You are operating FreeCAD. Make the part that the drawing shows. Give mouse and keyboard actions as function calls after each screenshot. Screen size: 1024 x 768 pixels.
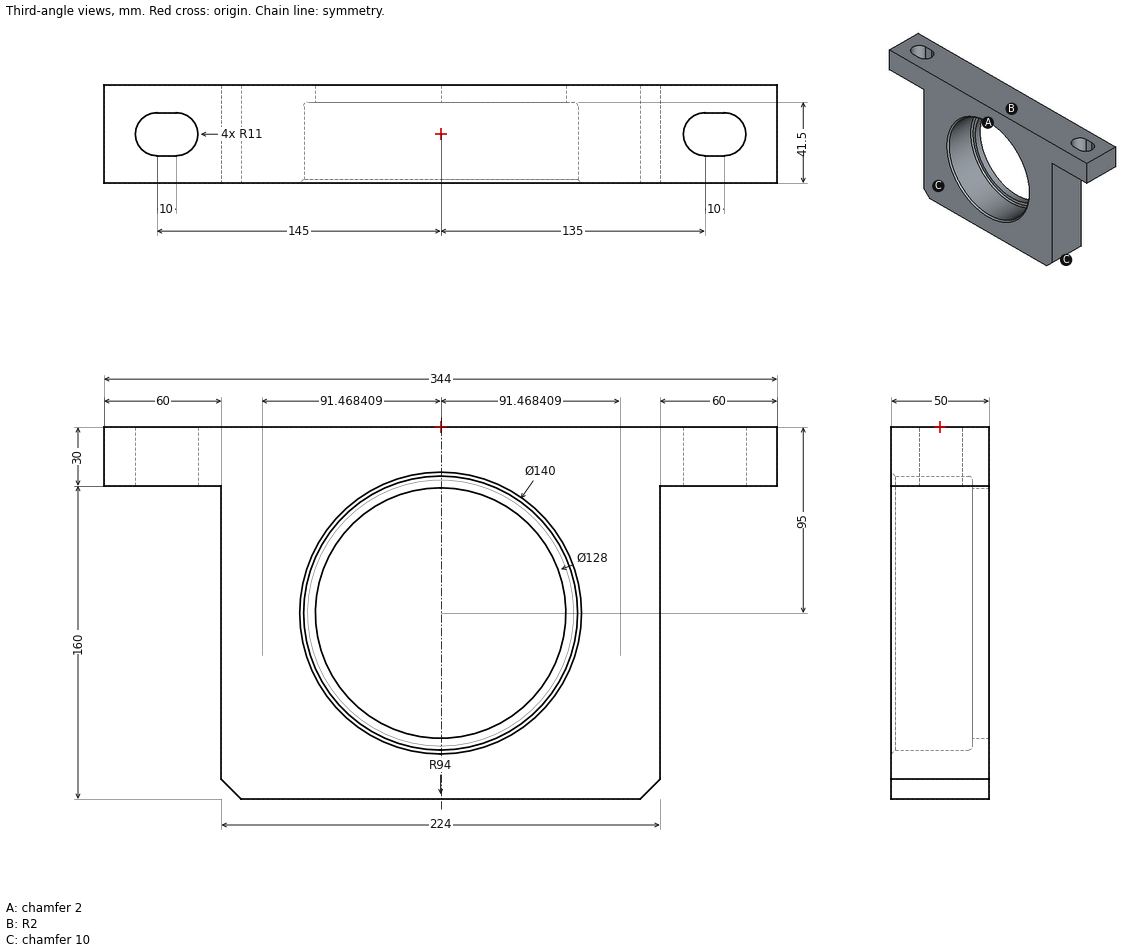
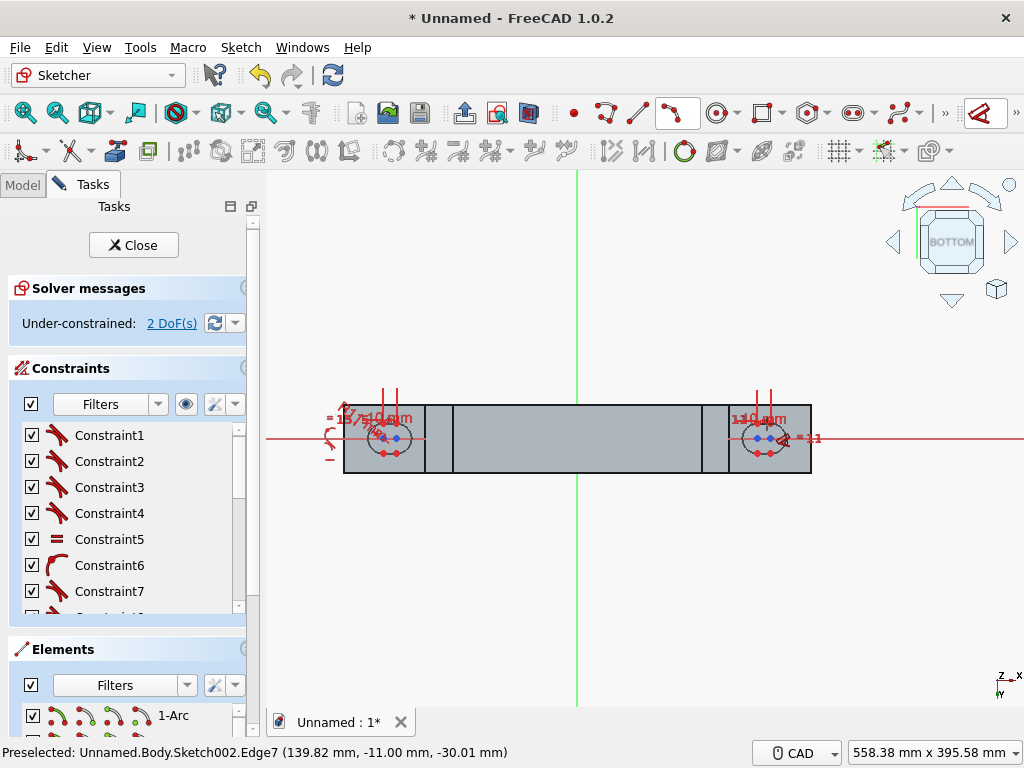
click(383, 424)
click(480, 390)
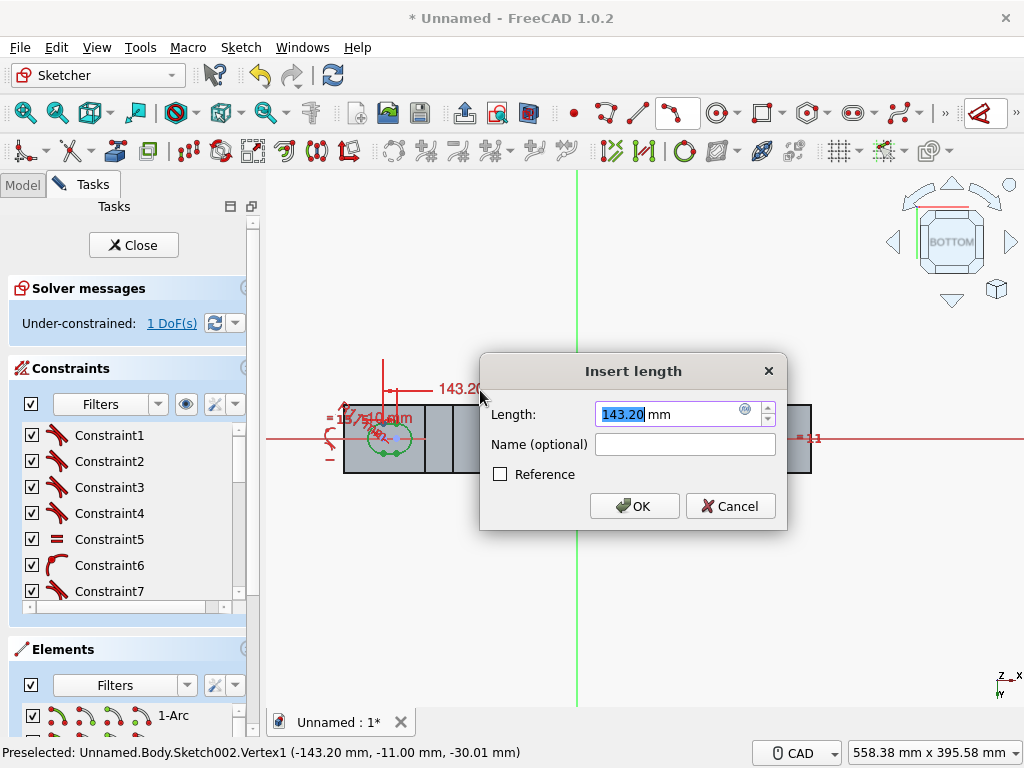
text(145)
key(Return)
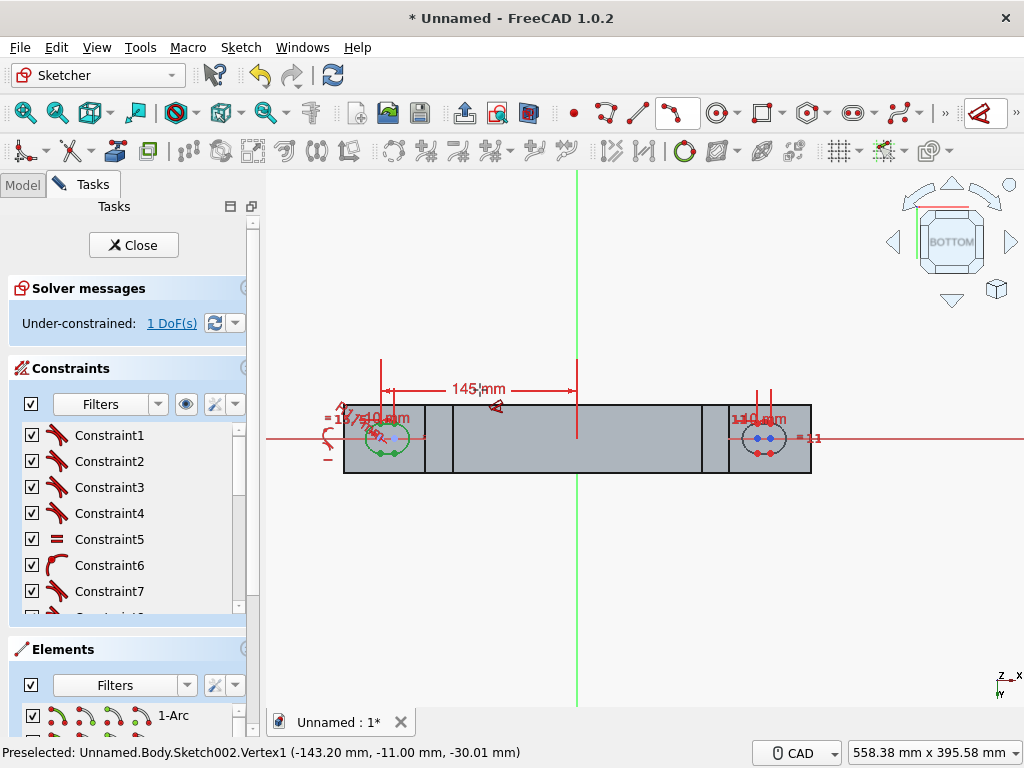
click(757, 424)
click(667, 390)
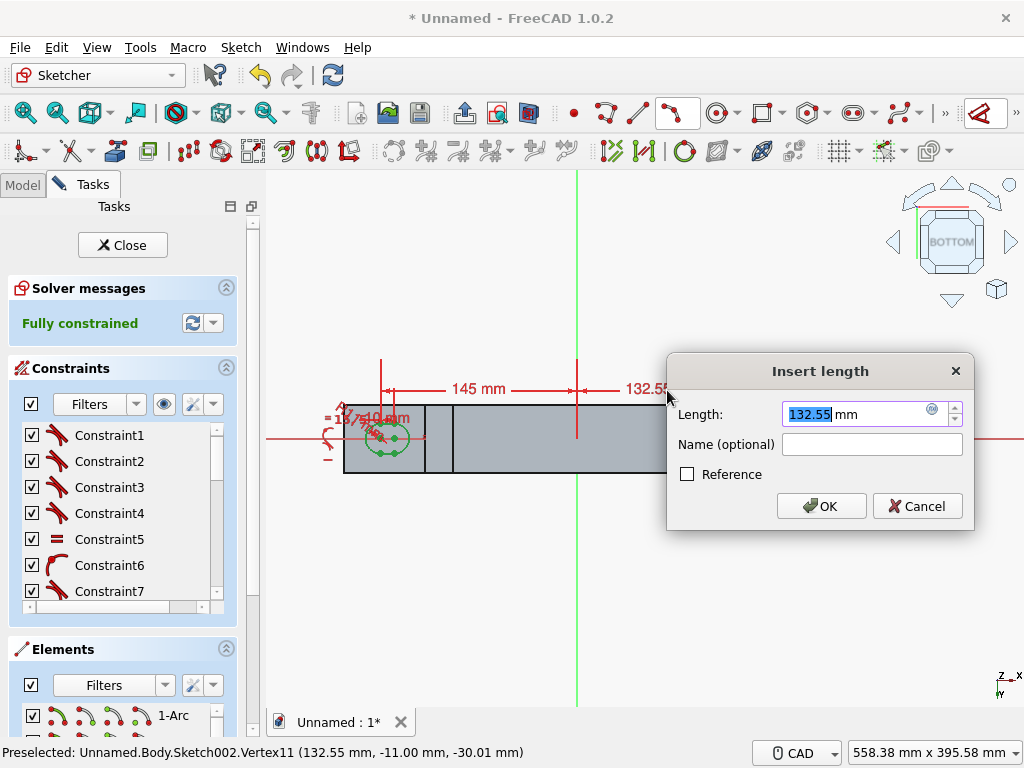
text(135)
key(Return)
key(Escape)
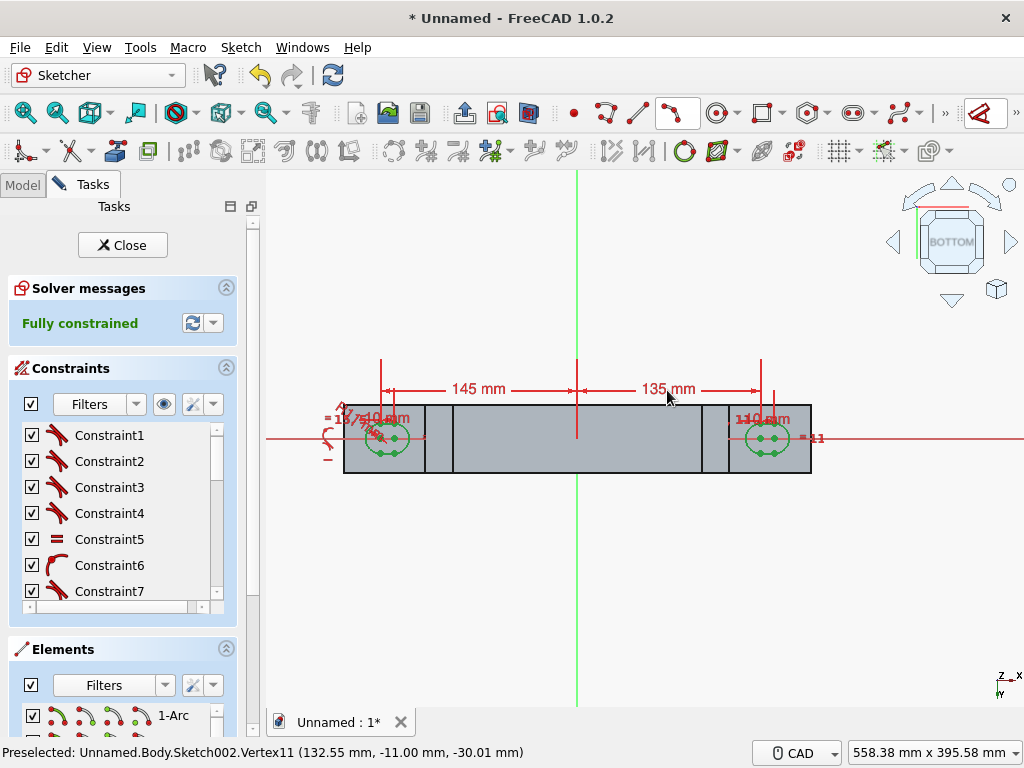
click(123, 245)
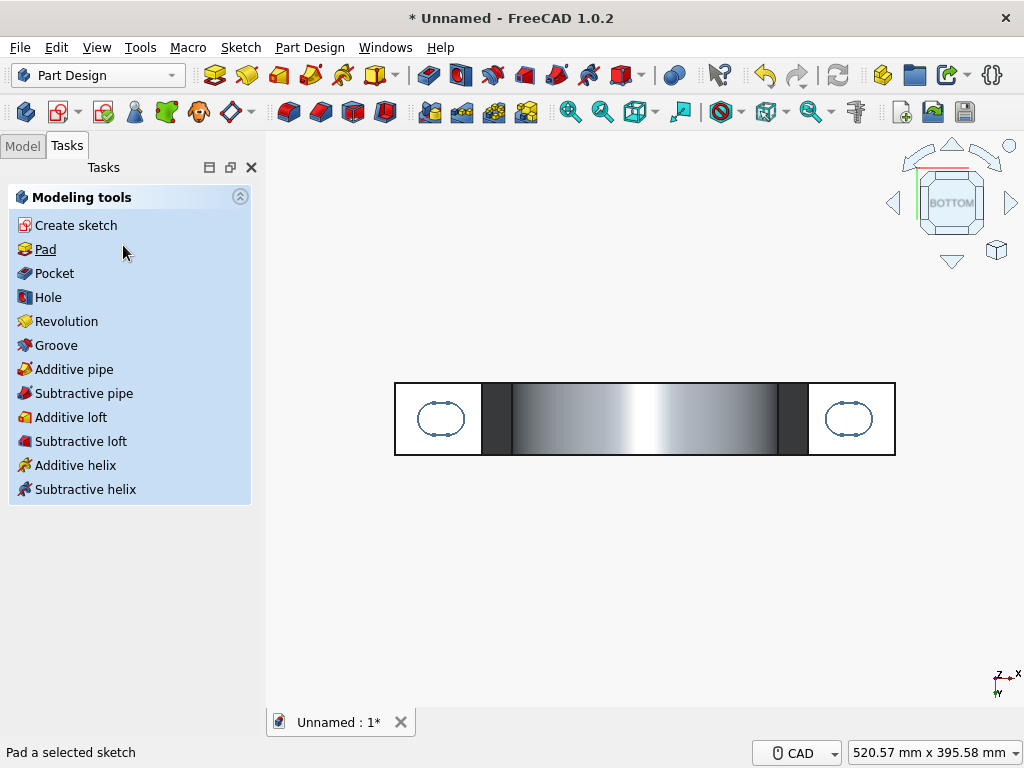
click(430, 76)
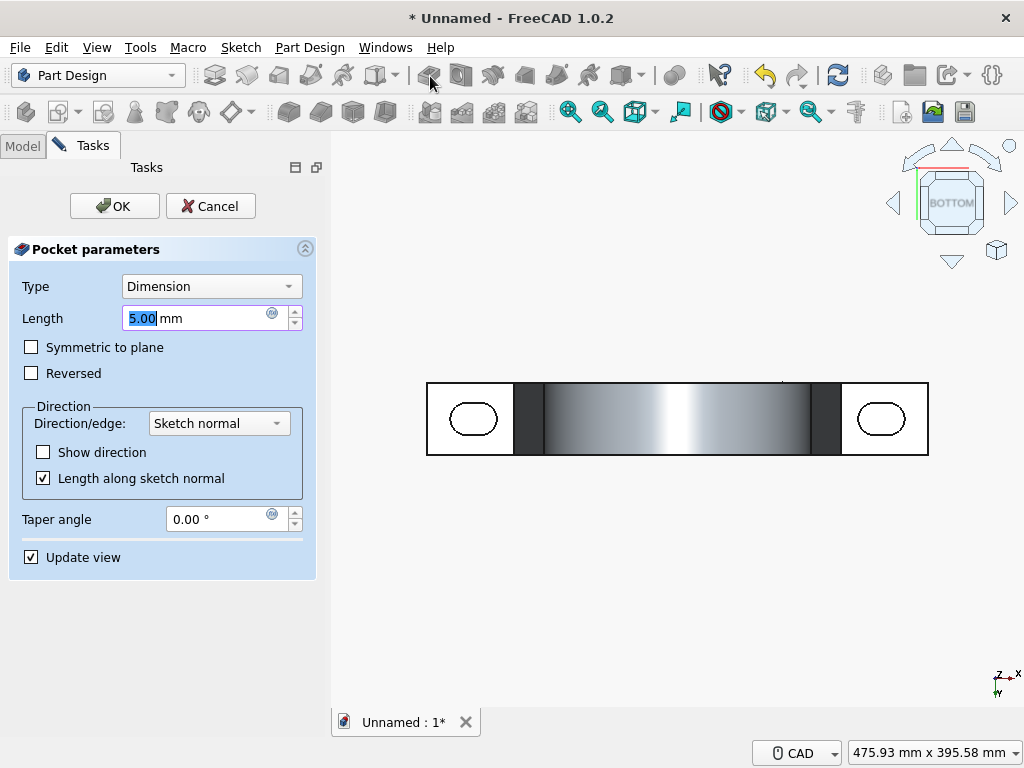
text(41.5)
key(Tab)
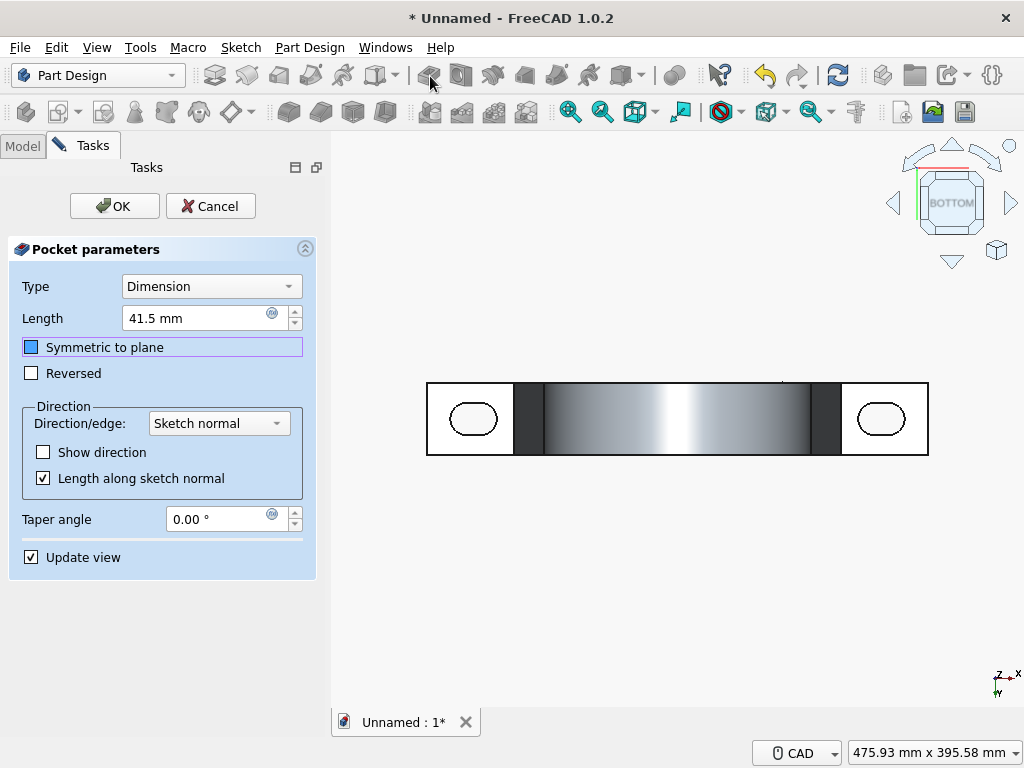
click(115, 206)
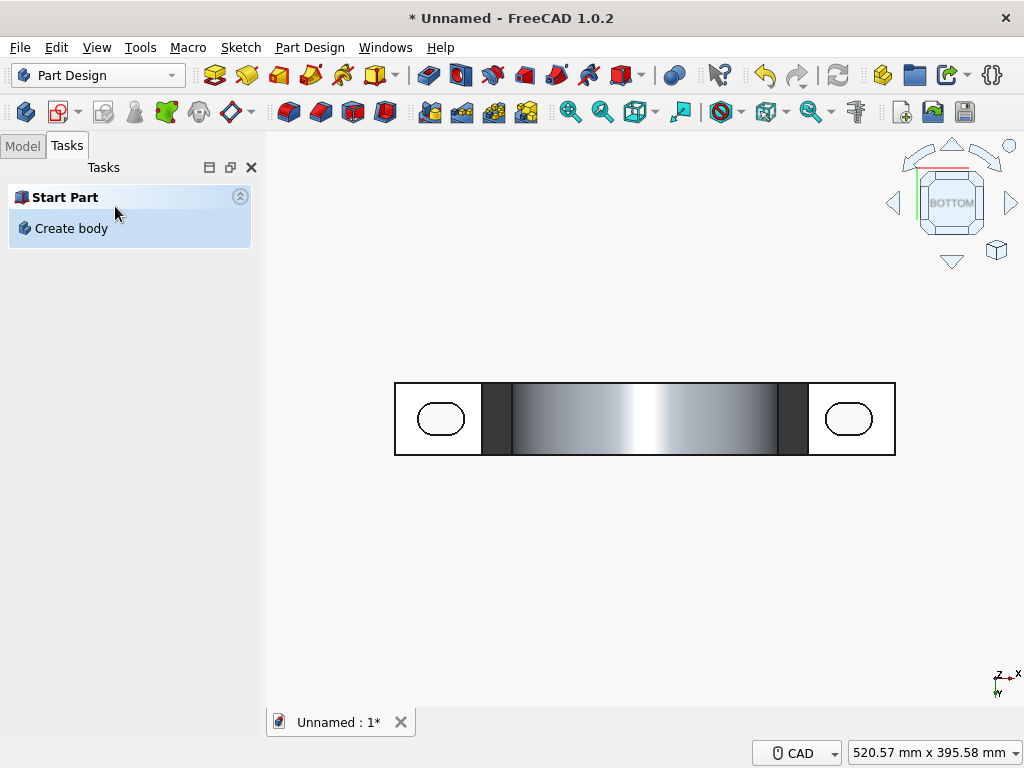
key(4)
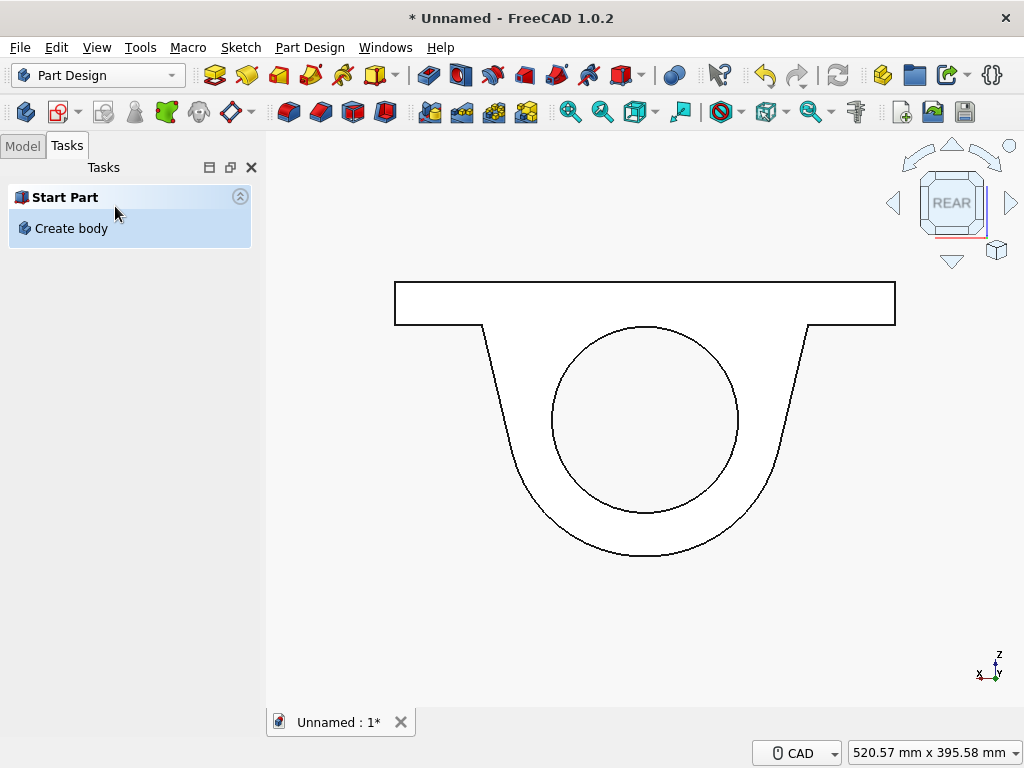
click(430, 300)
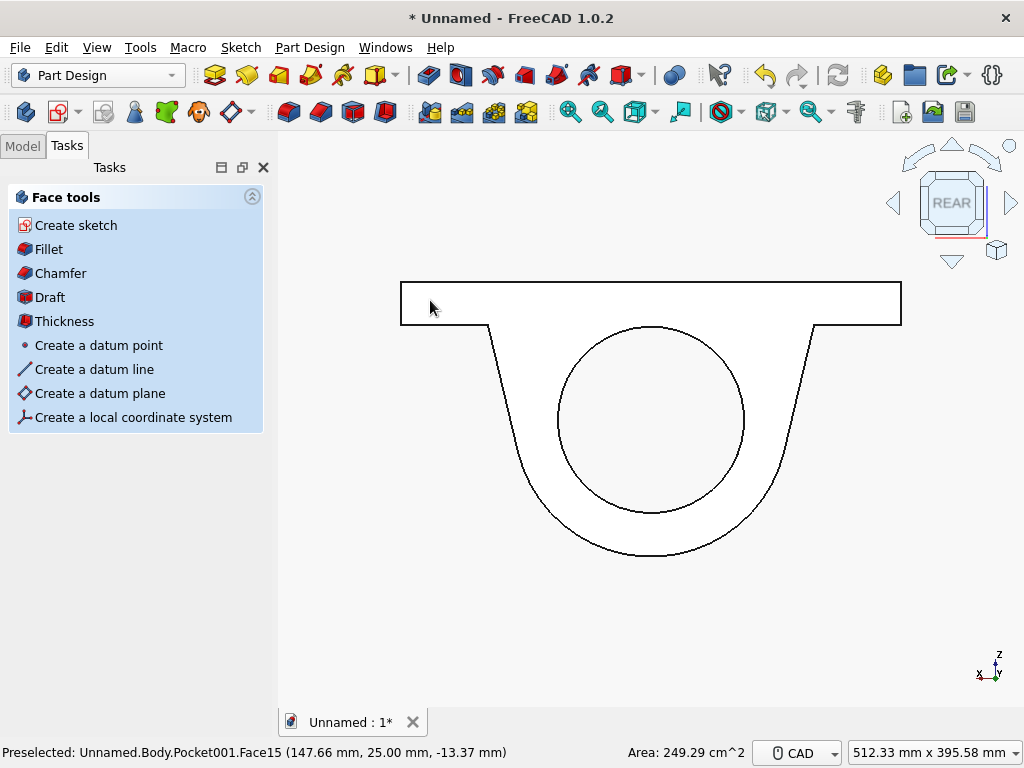
click(58, 112)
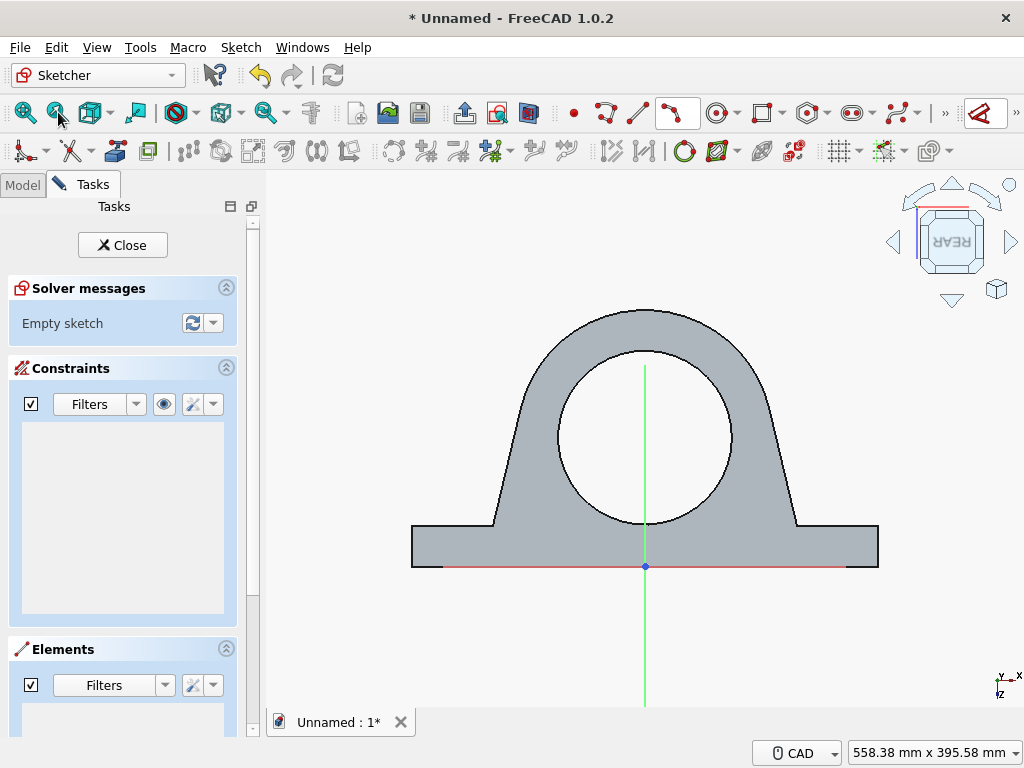
key(g)
key(m)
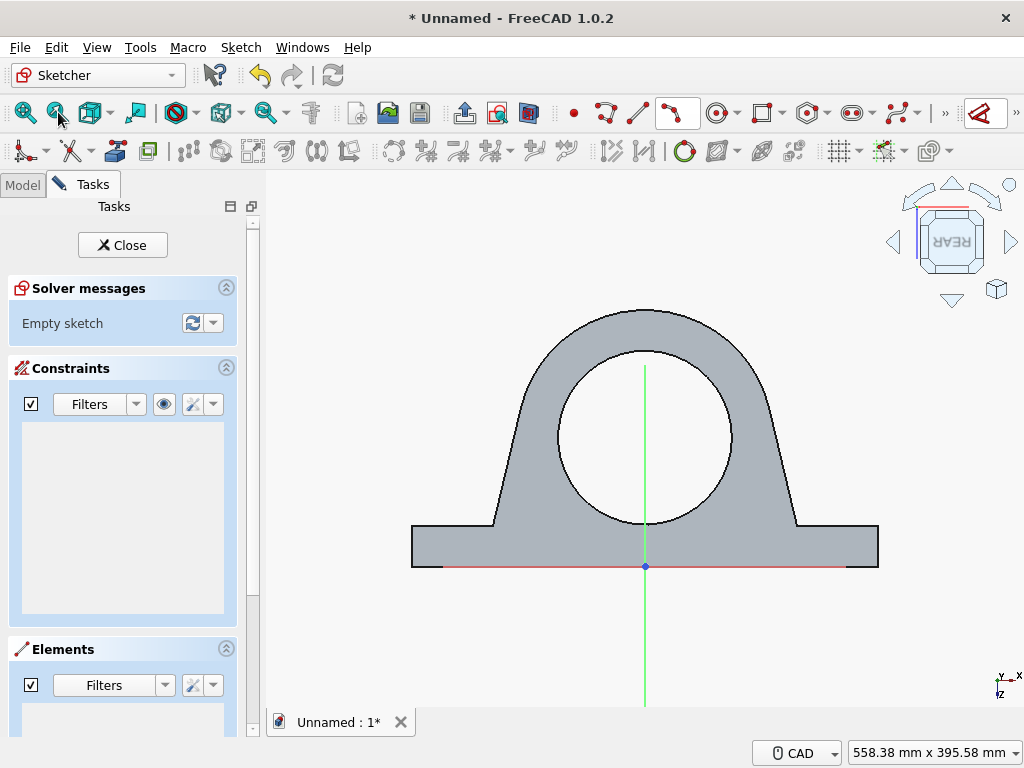
click(521, 408)
click(493, 526)
click(493, 309)
click(797, 309)
click(797, 526)
click(769, 408)
right_click(769, 408)